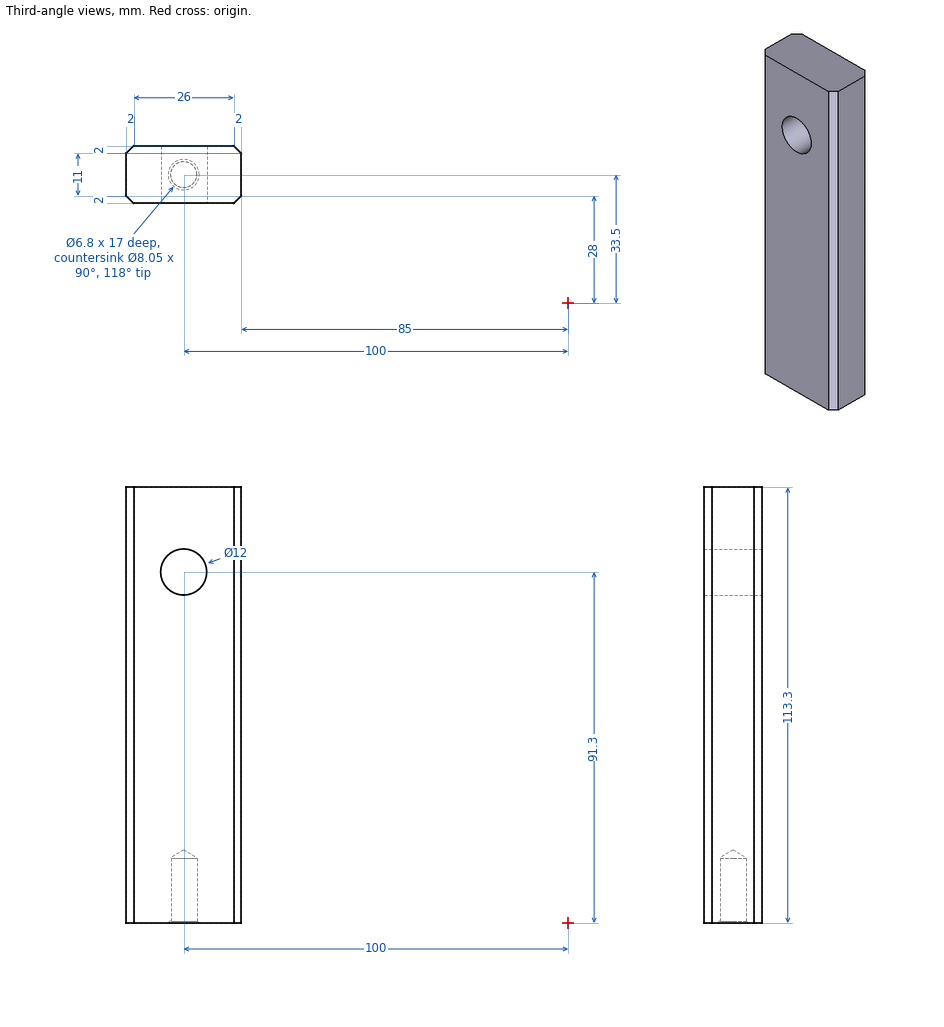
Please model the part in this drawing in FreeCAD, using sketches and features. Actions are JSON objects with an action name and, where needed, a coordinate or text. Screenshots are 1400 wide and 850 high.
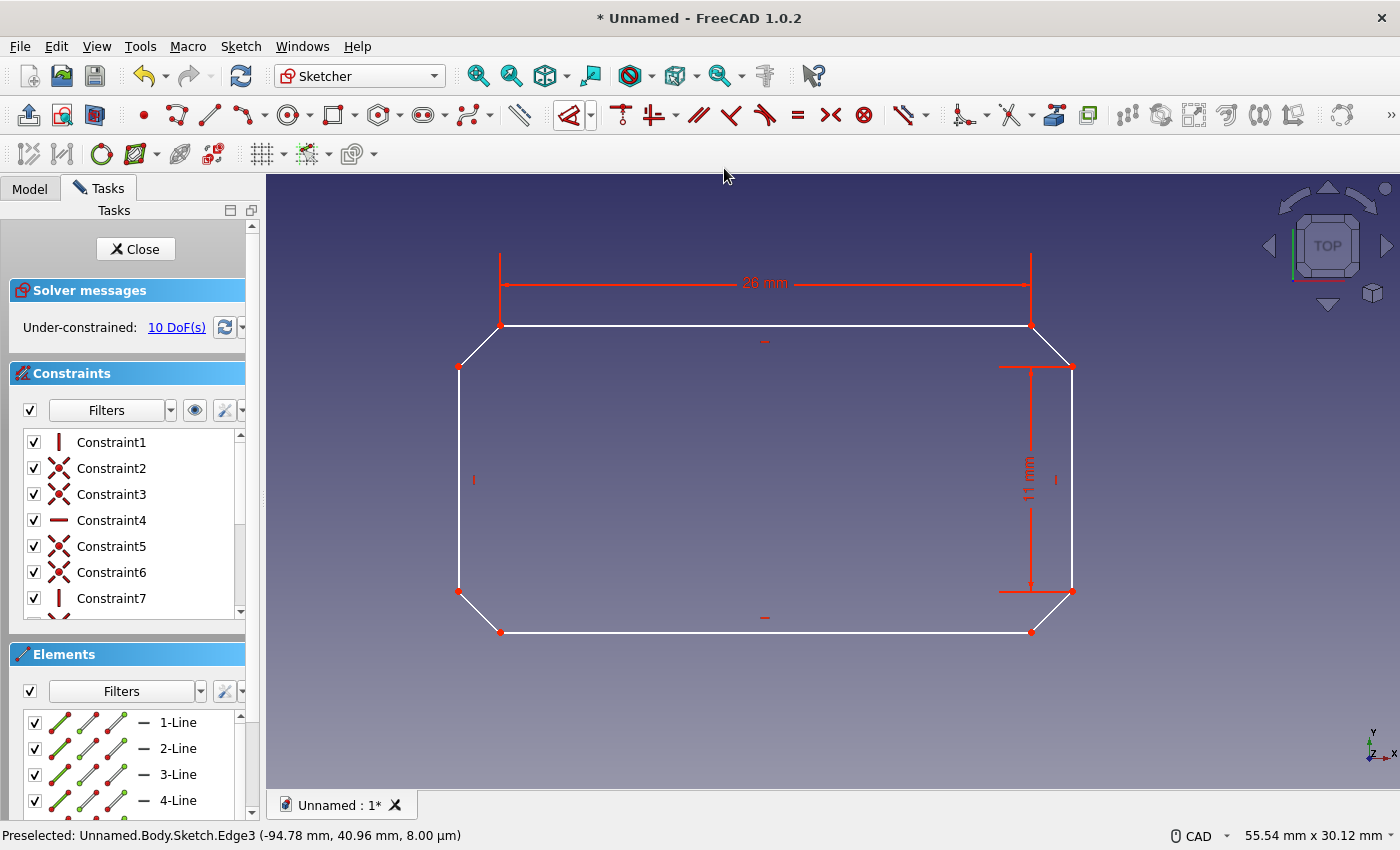
{"action": "left_click", "coordinate": [459, 434]}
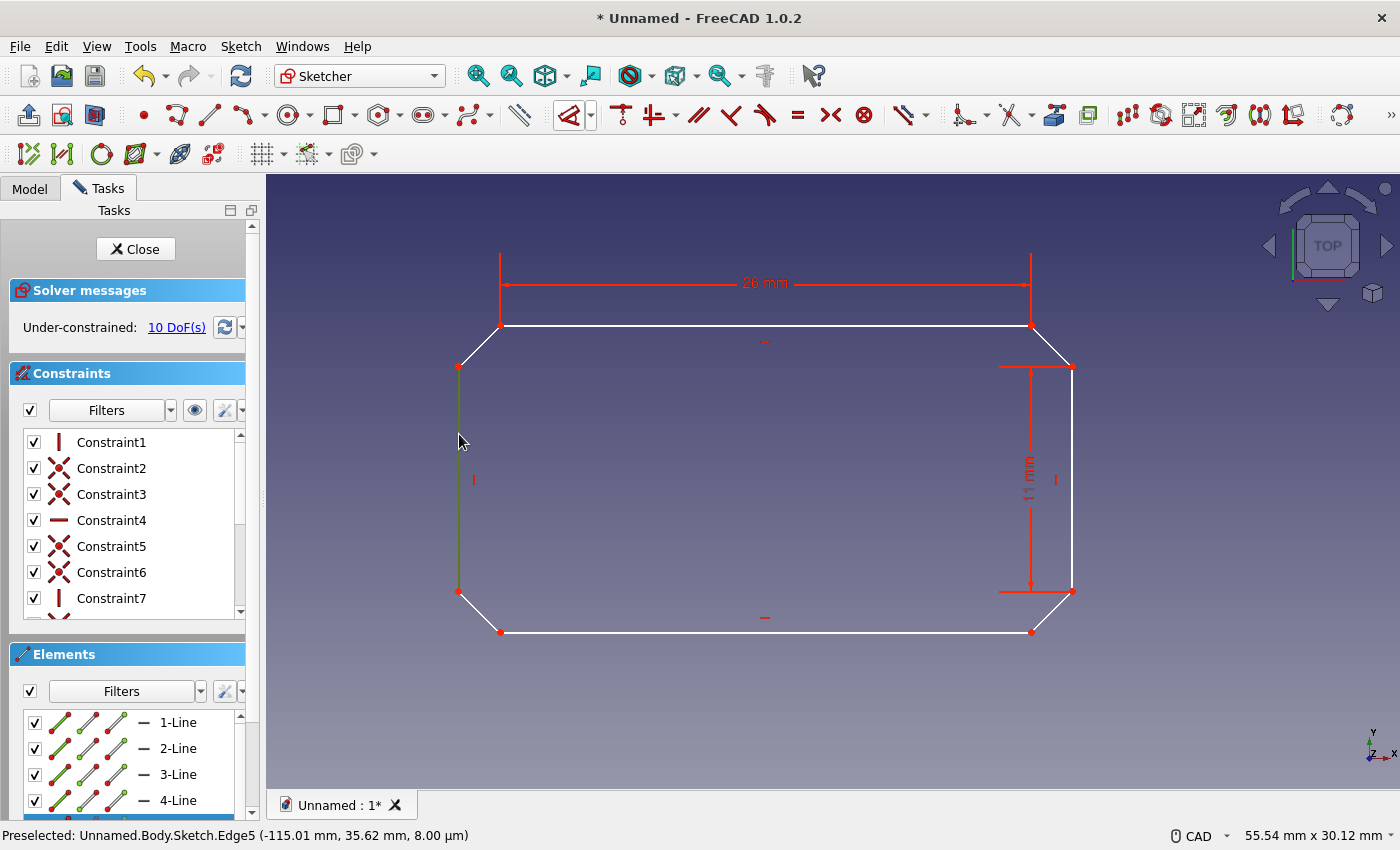
{"action": "key", "text": "i"}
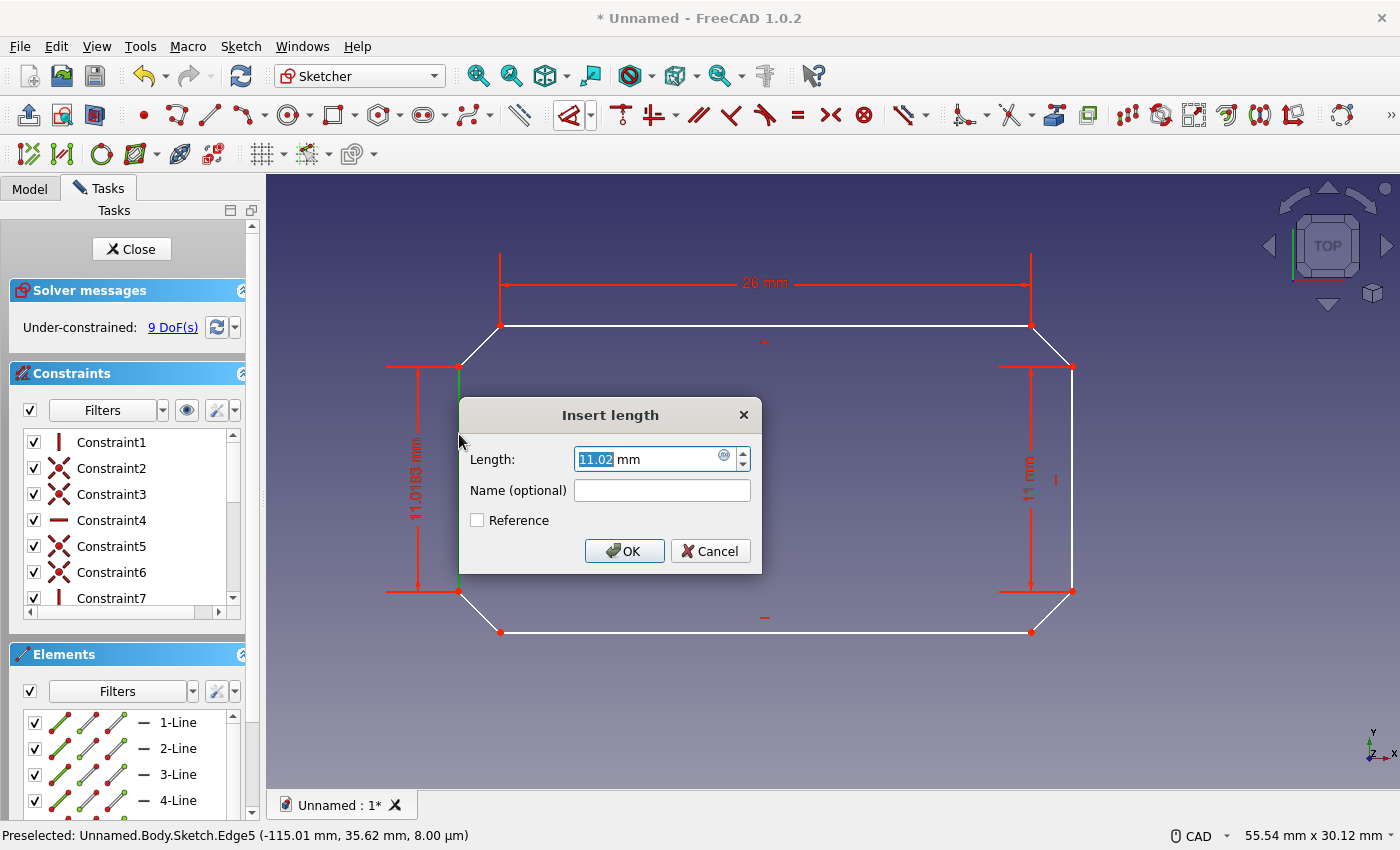
{"action": "type", "text": "11"}
{"action": "key", "text": "Return"}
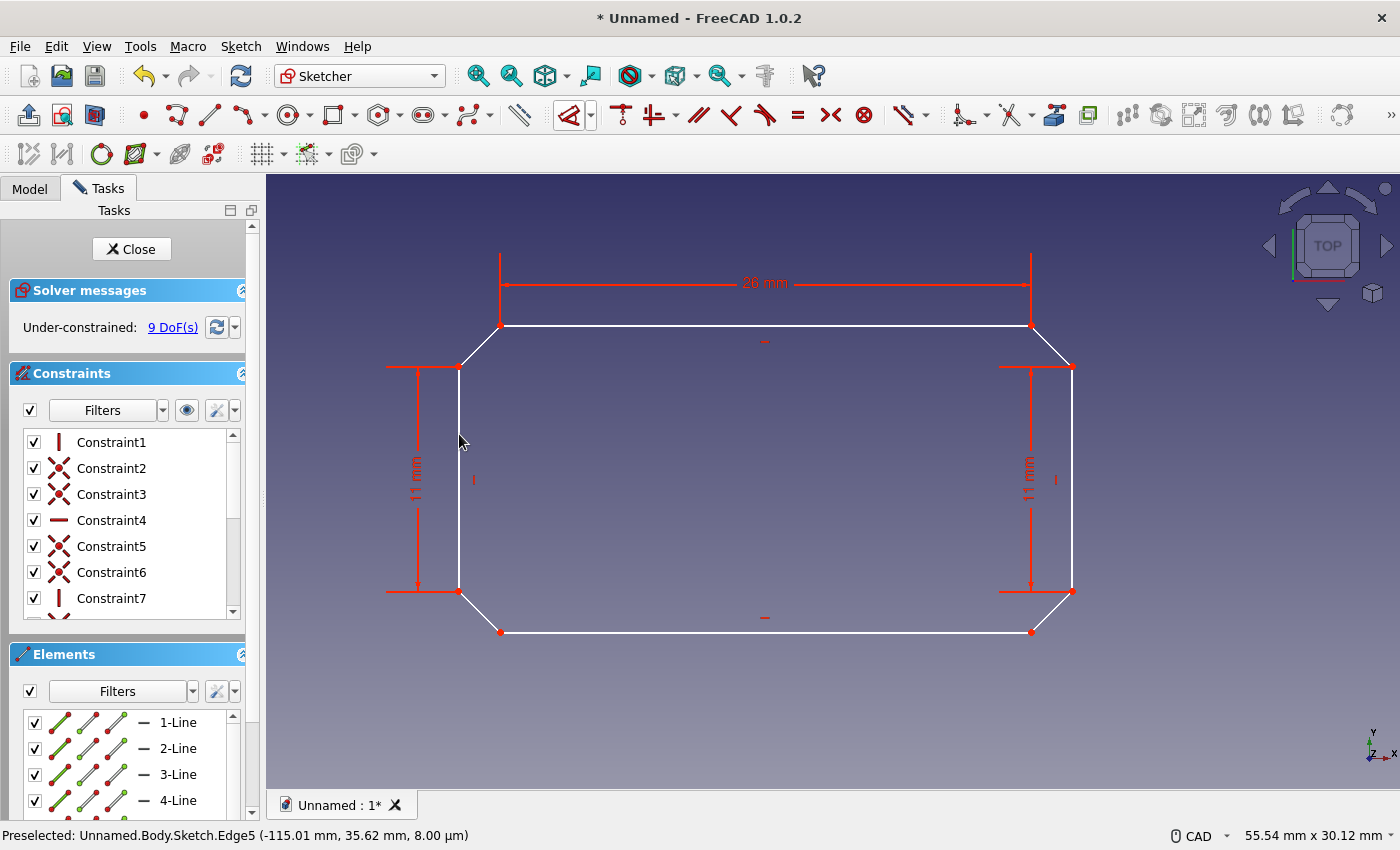
{"action": "left_click", "coordinate": [659, 633]}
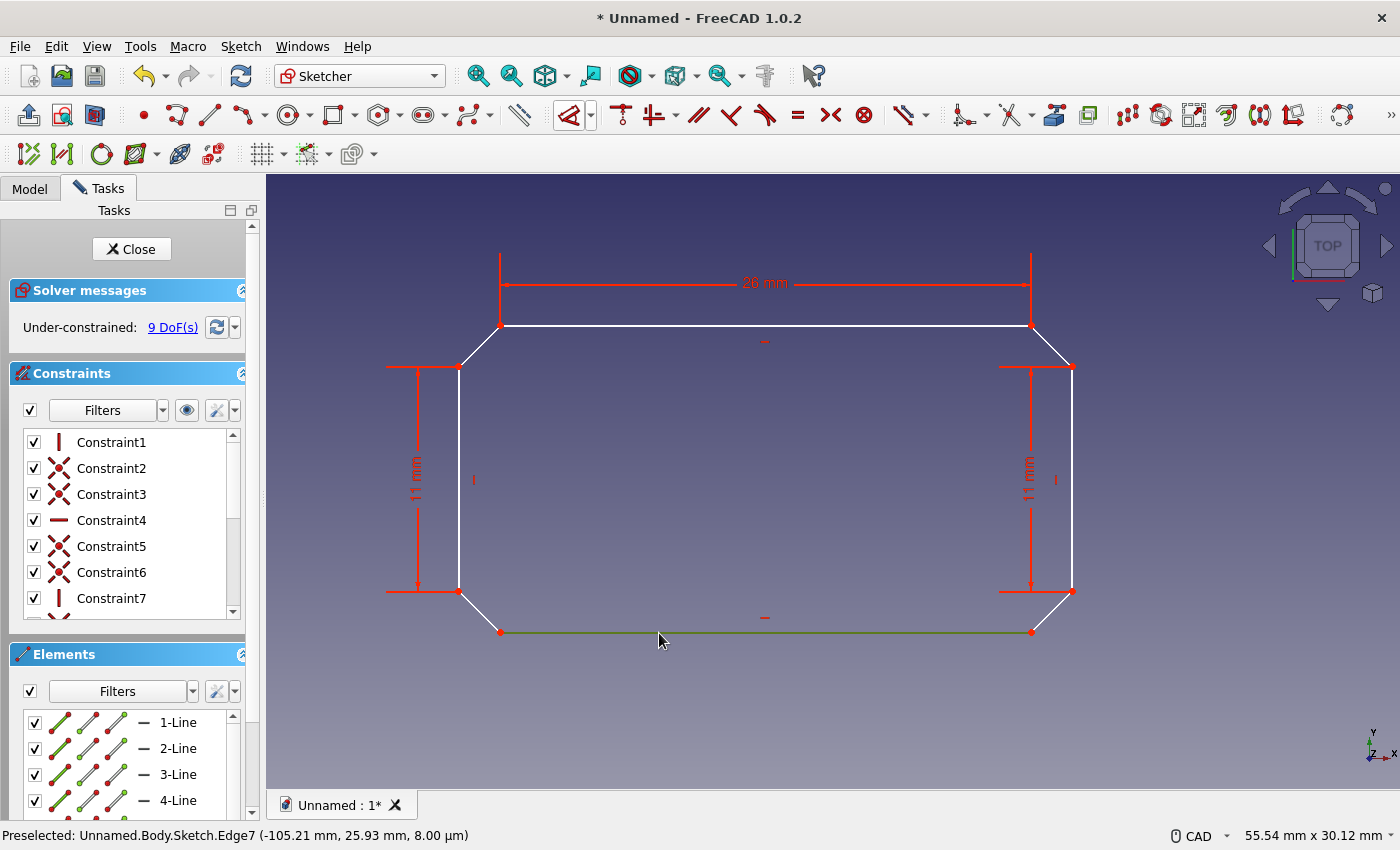
{"action": "left_click", "coordinate": [590, 116]}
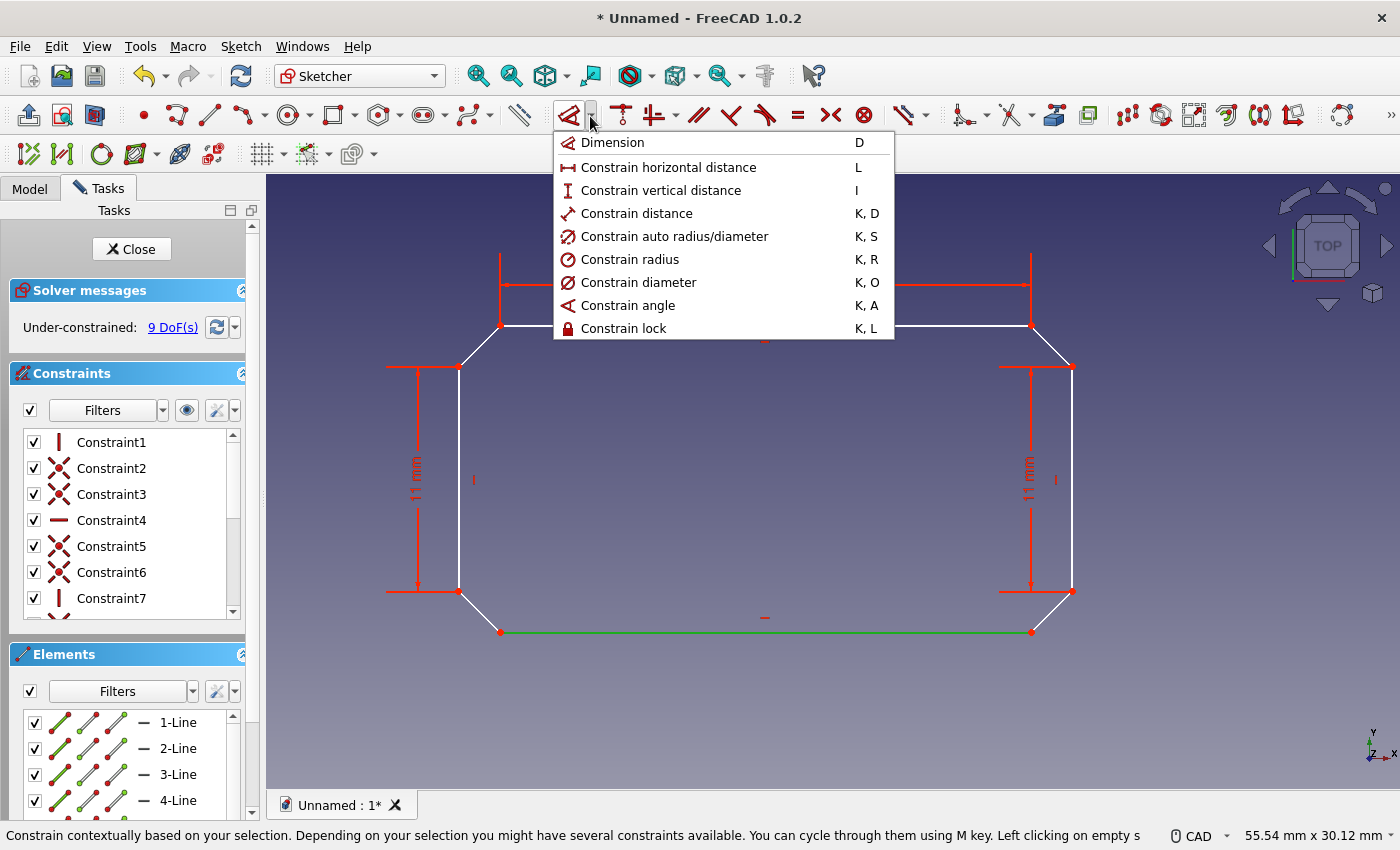
{"action": "left_click", "coordinate": [724, 168]}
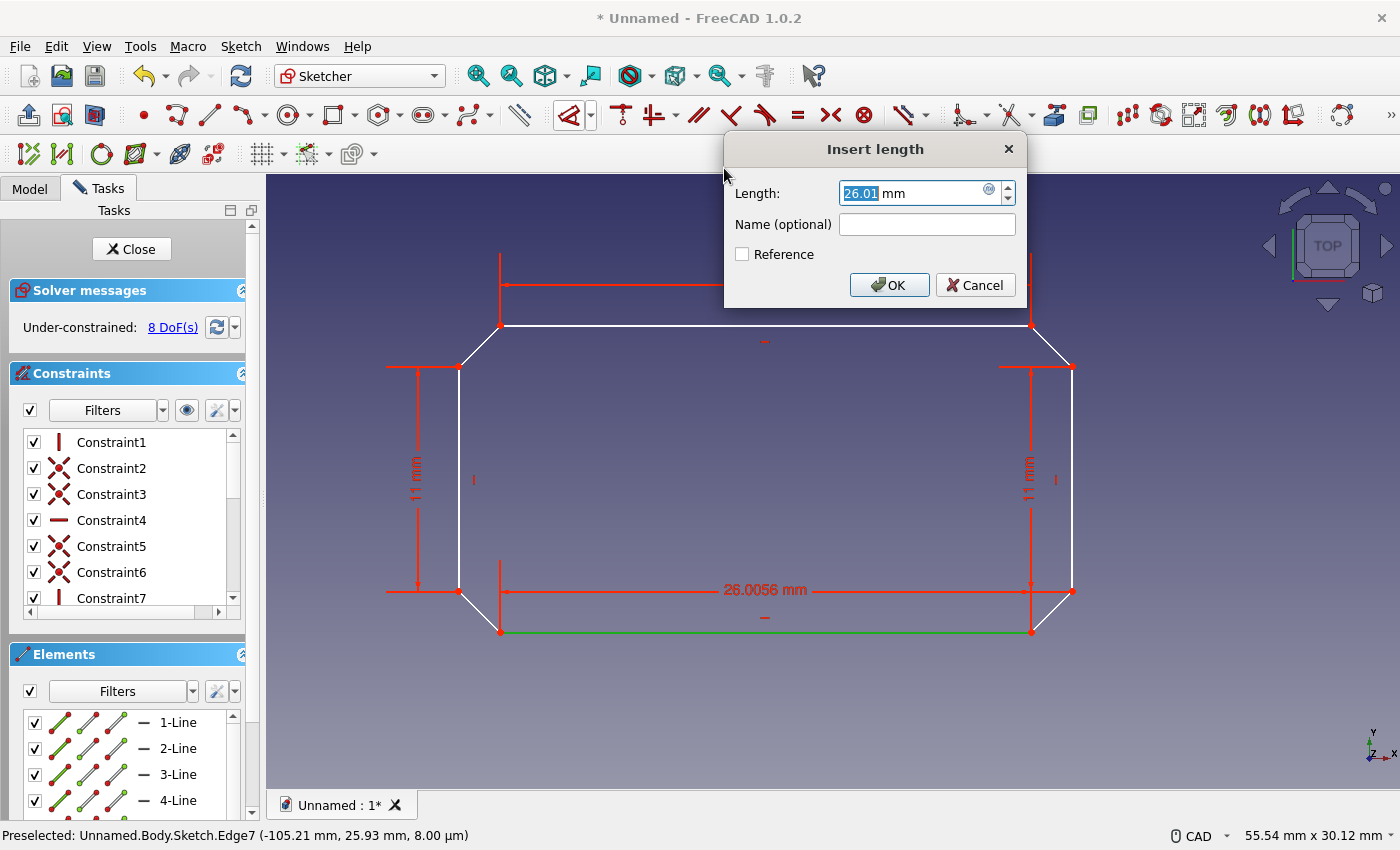
{"action": "type", "text": "26"}
{"action": "key", "text": "Return"}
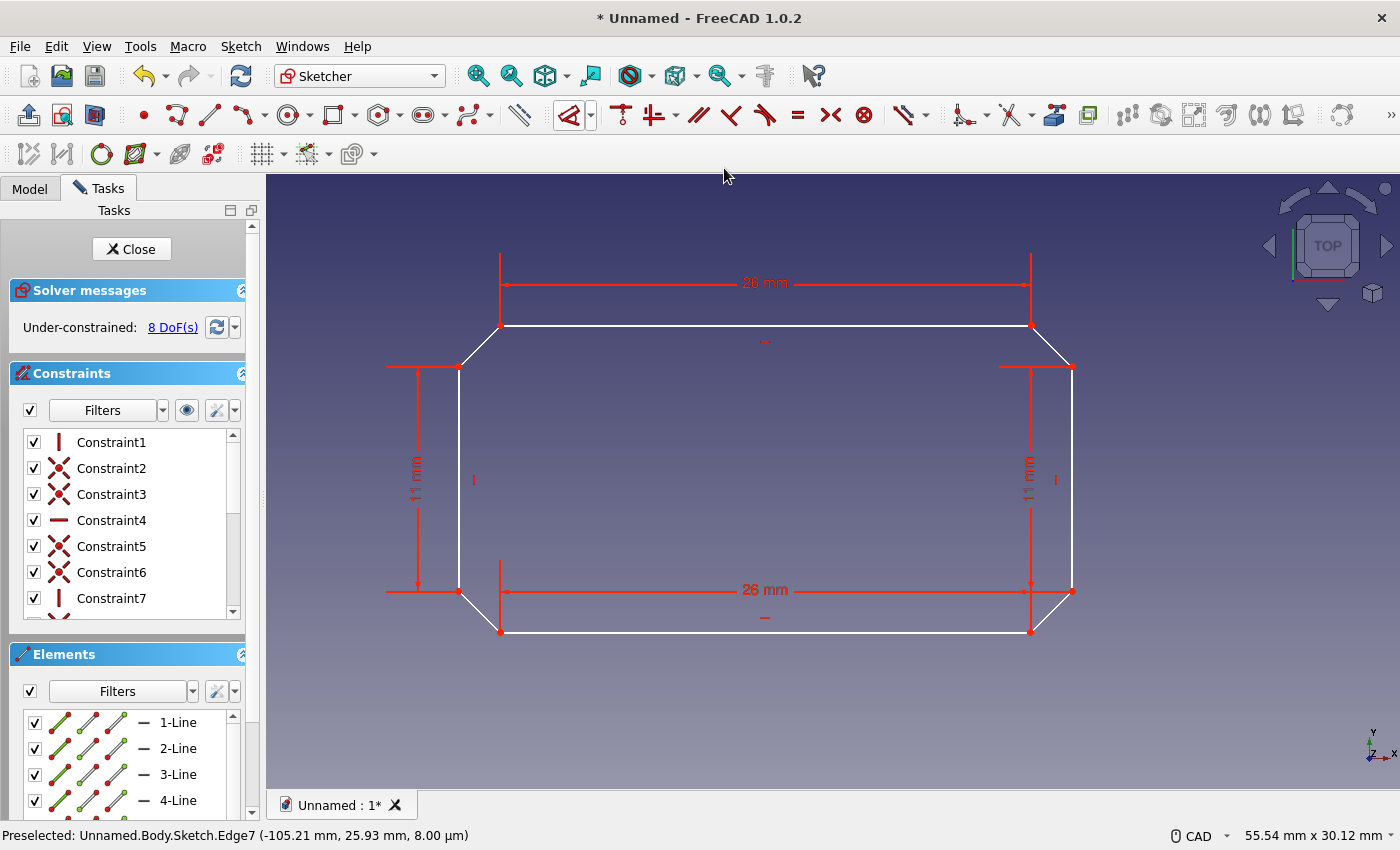
{"action": "left_click", "coordinate": [1060, 355]}